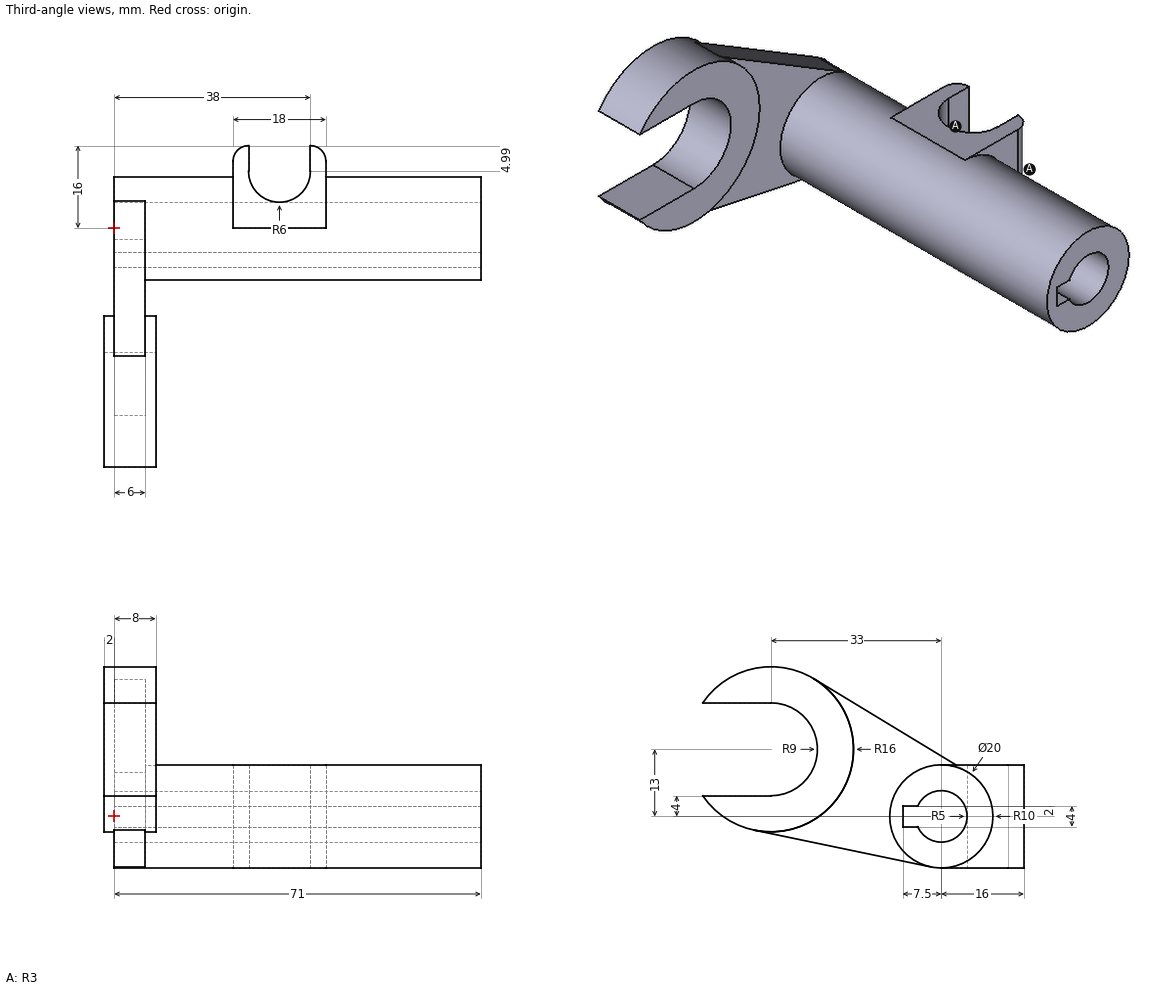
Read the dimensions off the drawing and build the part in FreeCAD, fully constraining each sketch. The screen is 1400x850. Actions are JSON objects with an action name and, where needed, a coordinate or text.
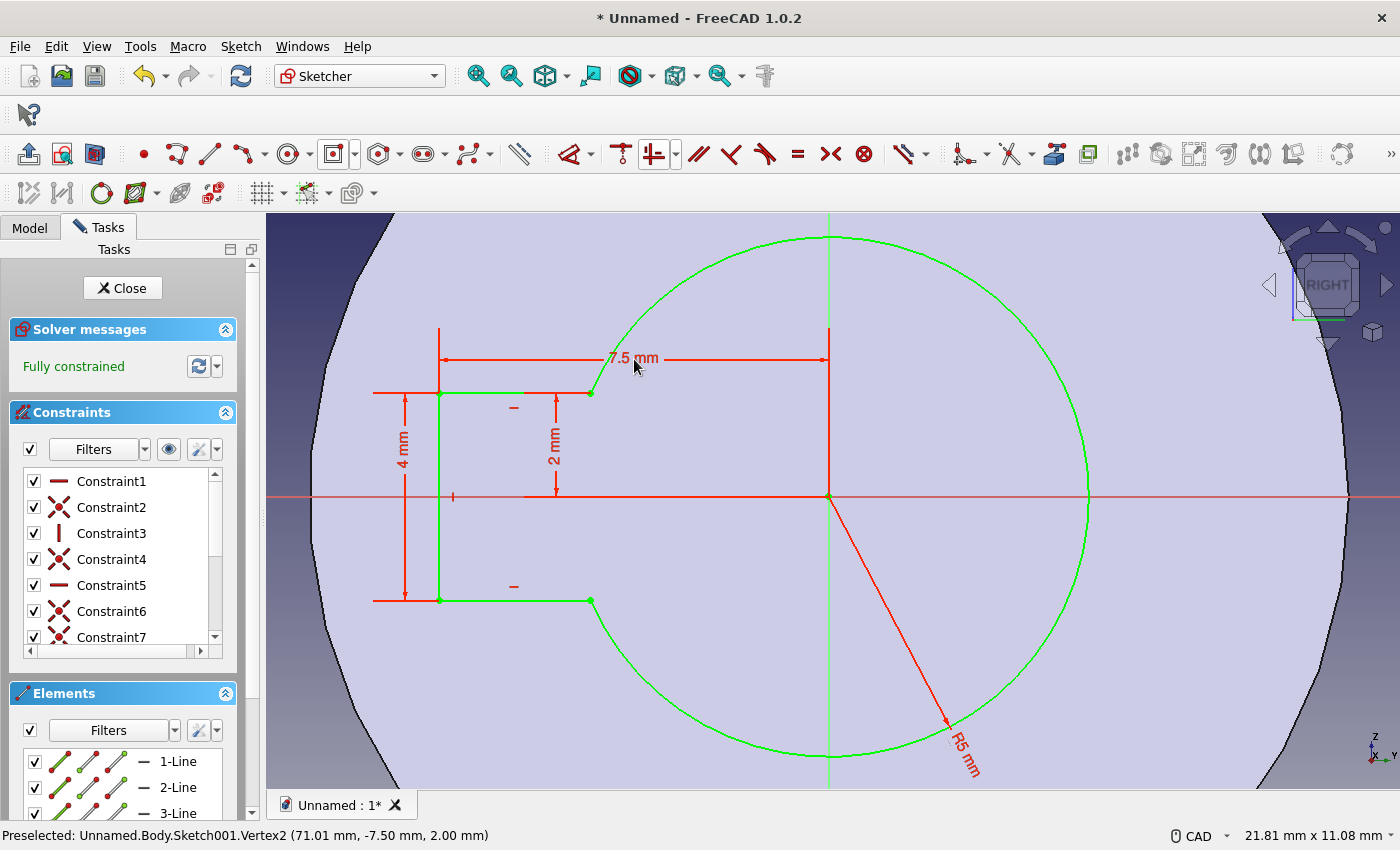
{"action": "left_click", "coordinate": [123, 288]}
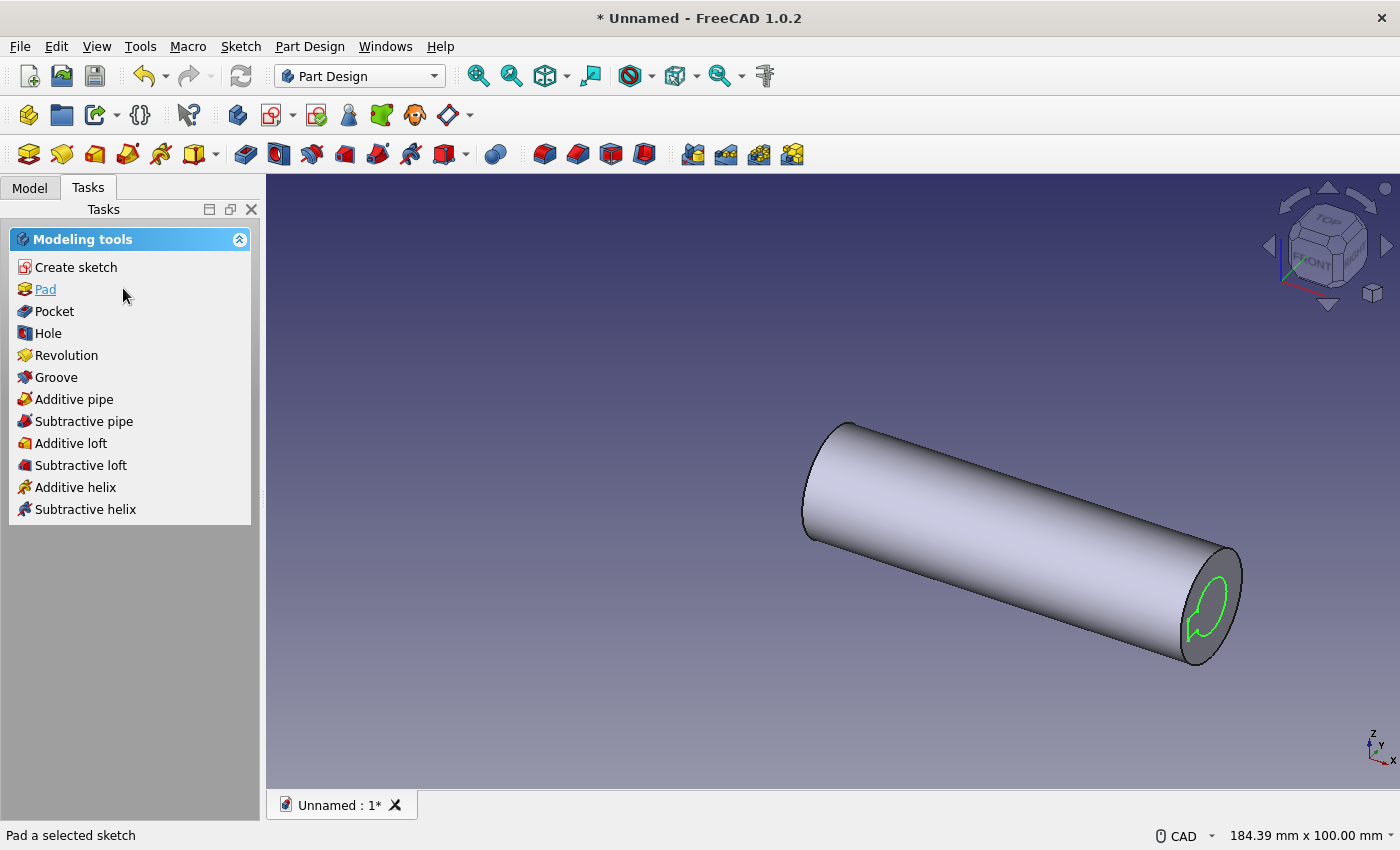
{"action": "left_click", "coordinate": [246, 154]}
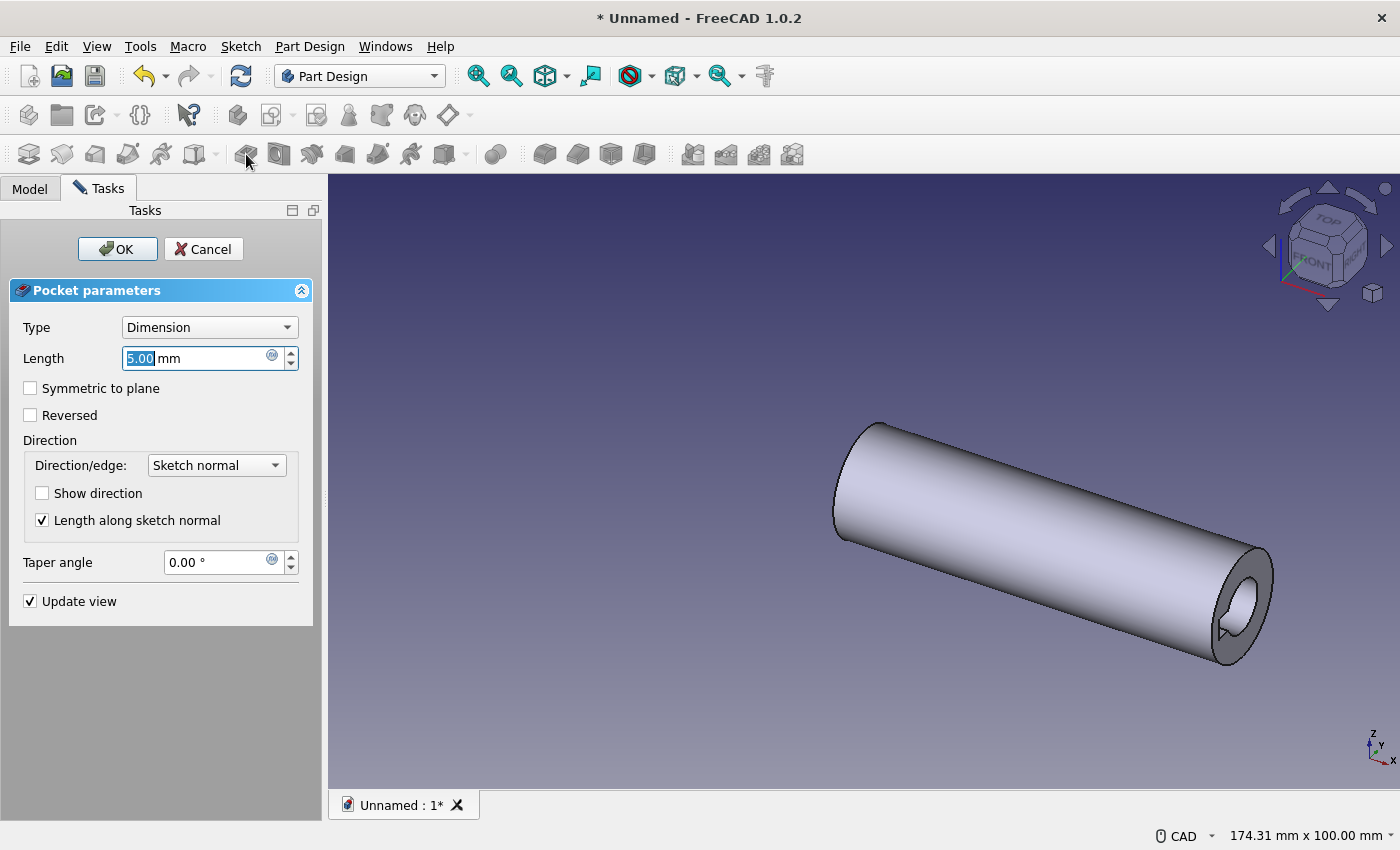
{"action": "left_click", "coordinate": [210, 328]}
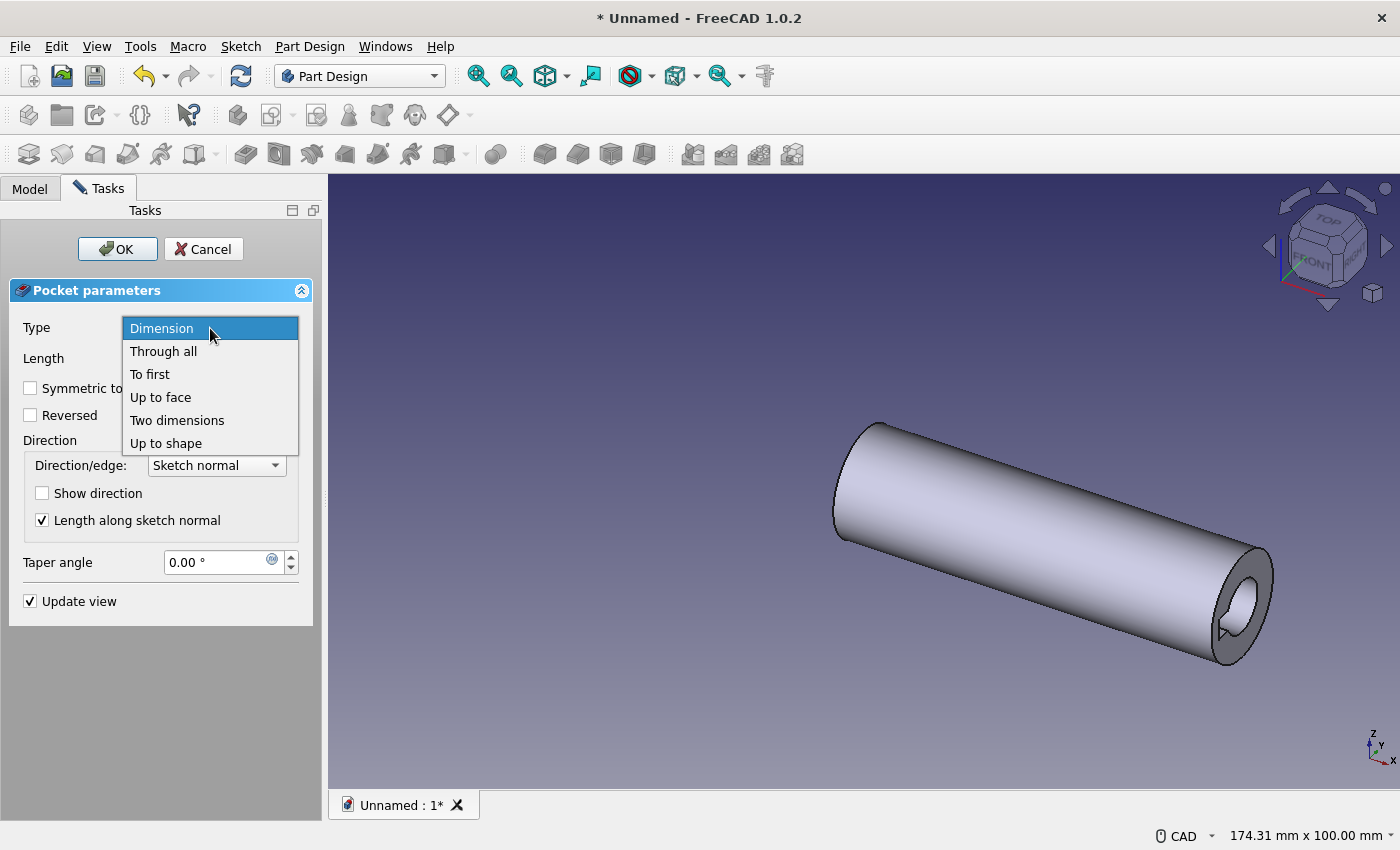
{"action": "left_click", "coordinate": [208, 374]}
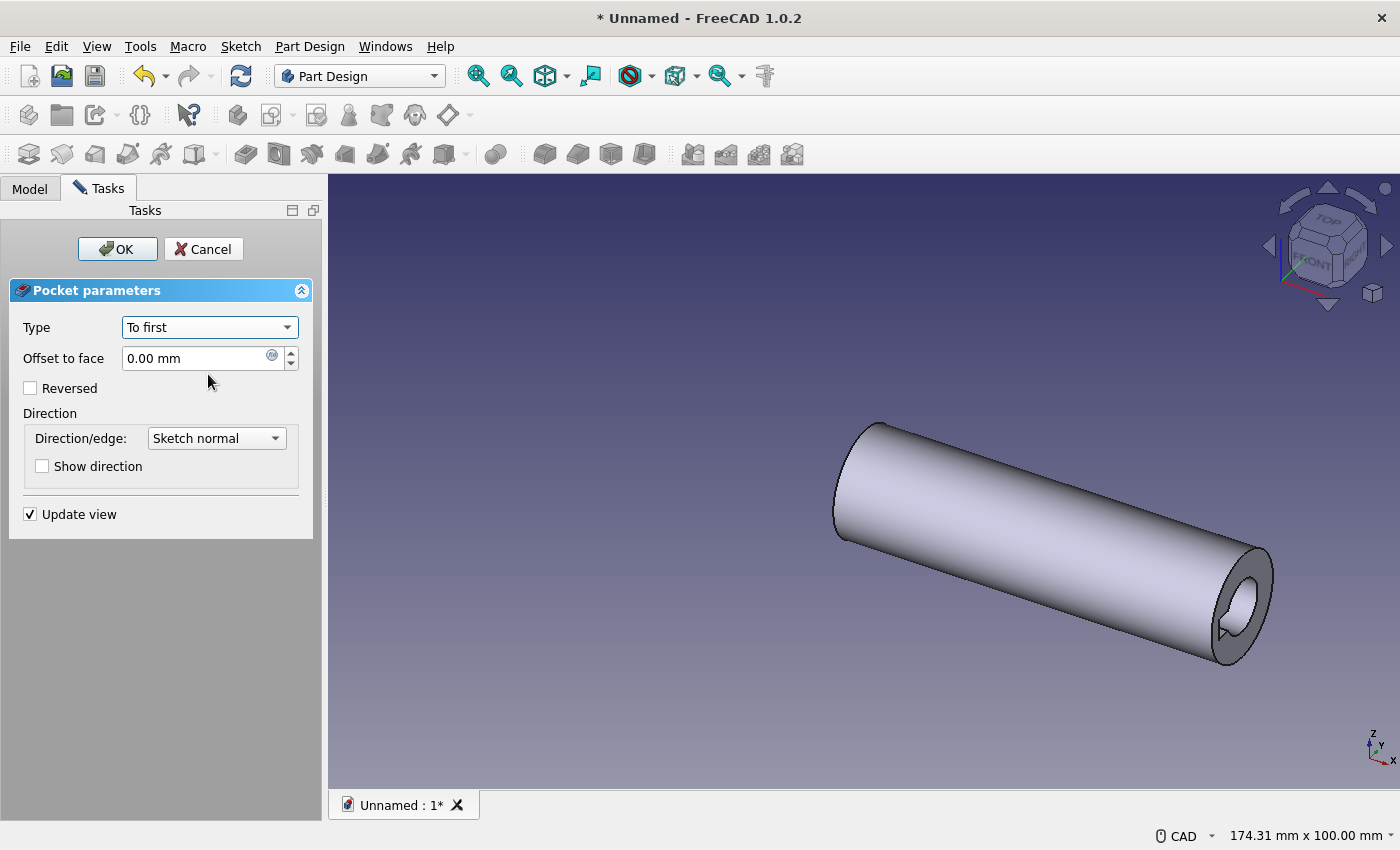
{"action": "left_click", "coordinate": [118, 249]}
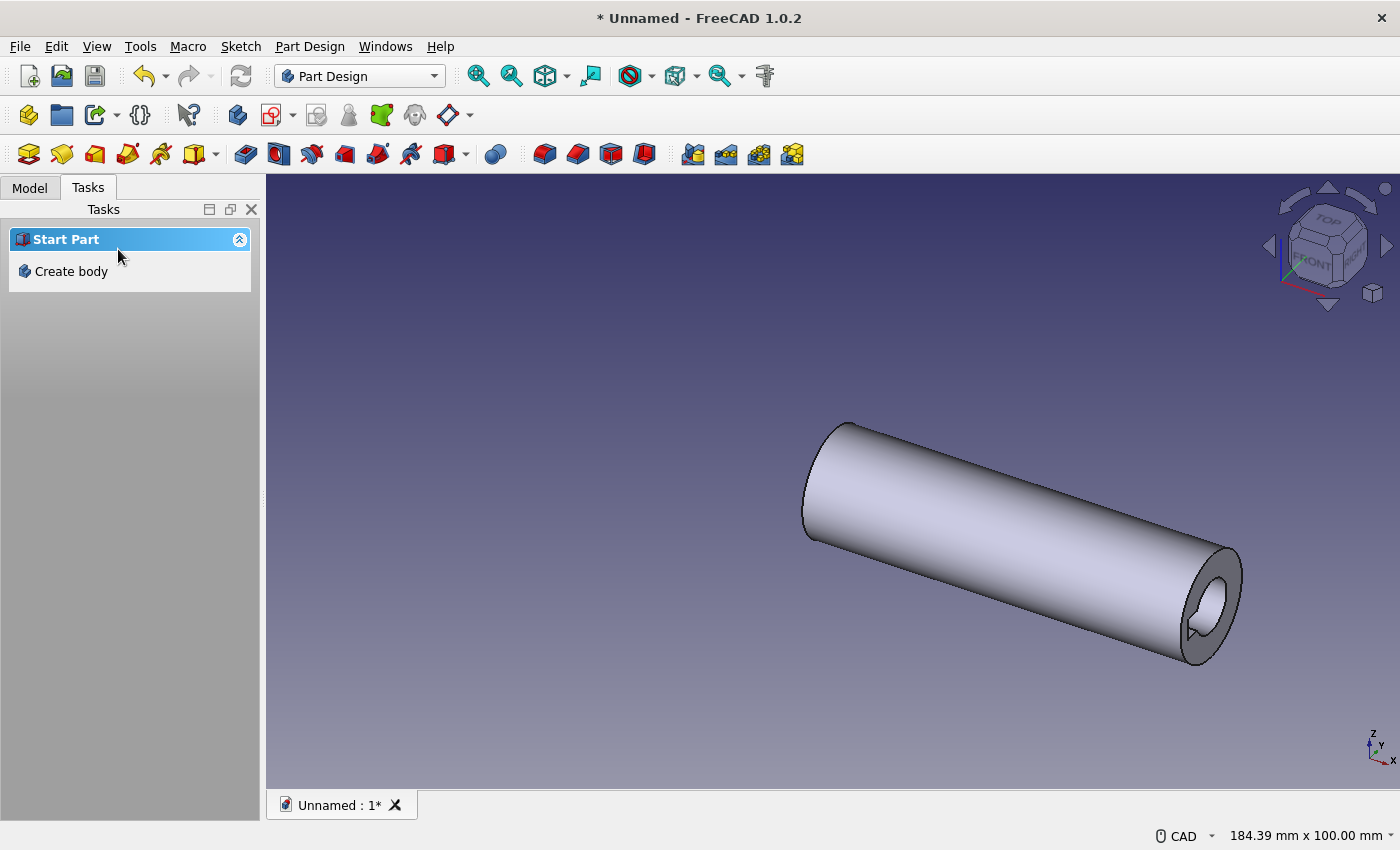
{"action": "left_click", "coordinate": [30, 188]}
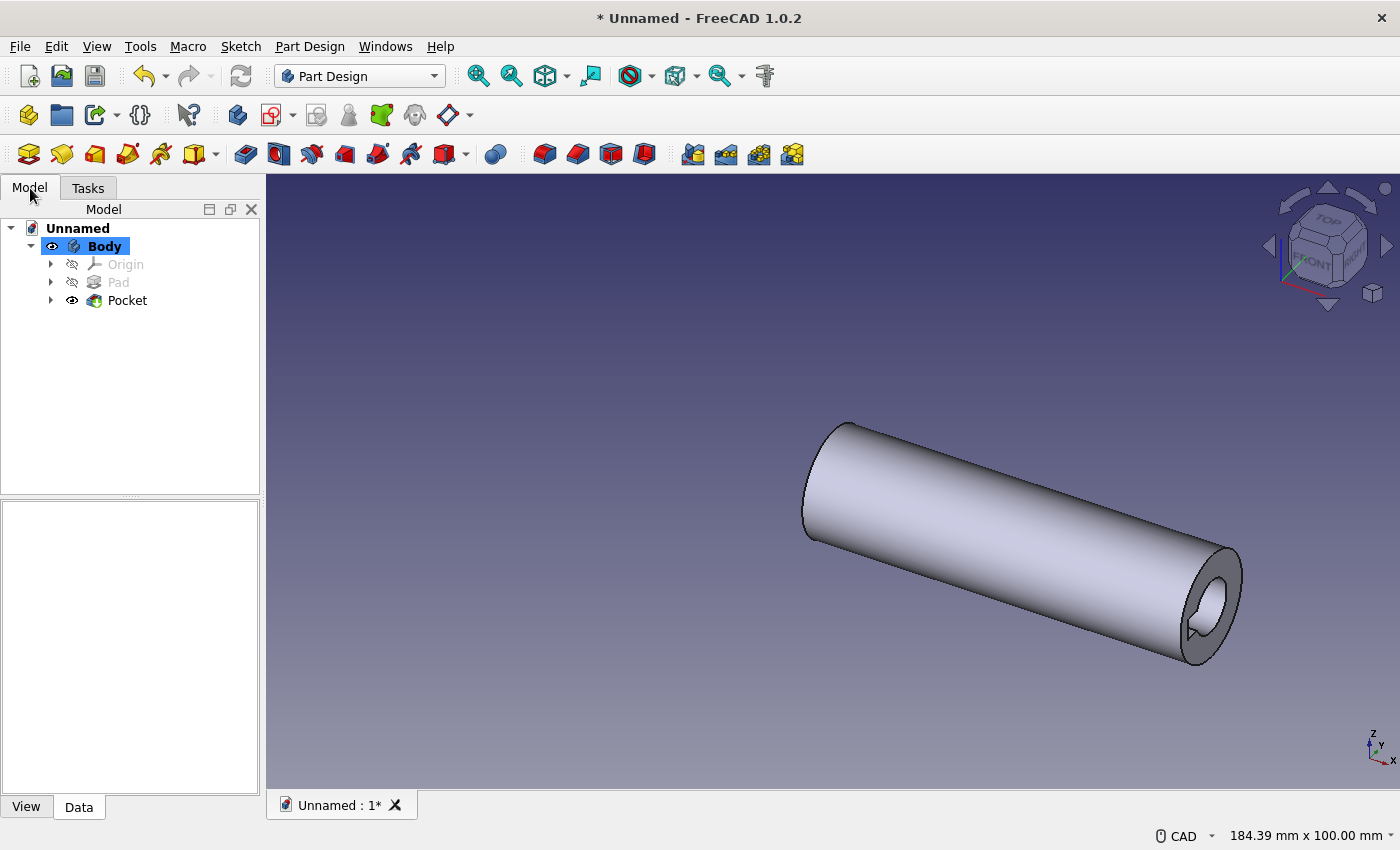
{"action": "left_click", "coordinate": [51, 264]}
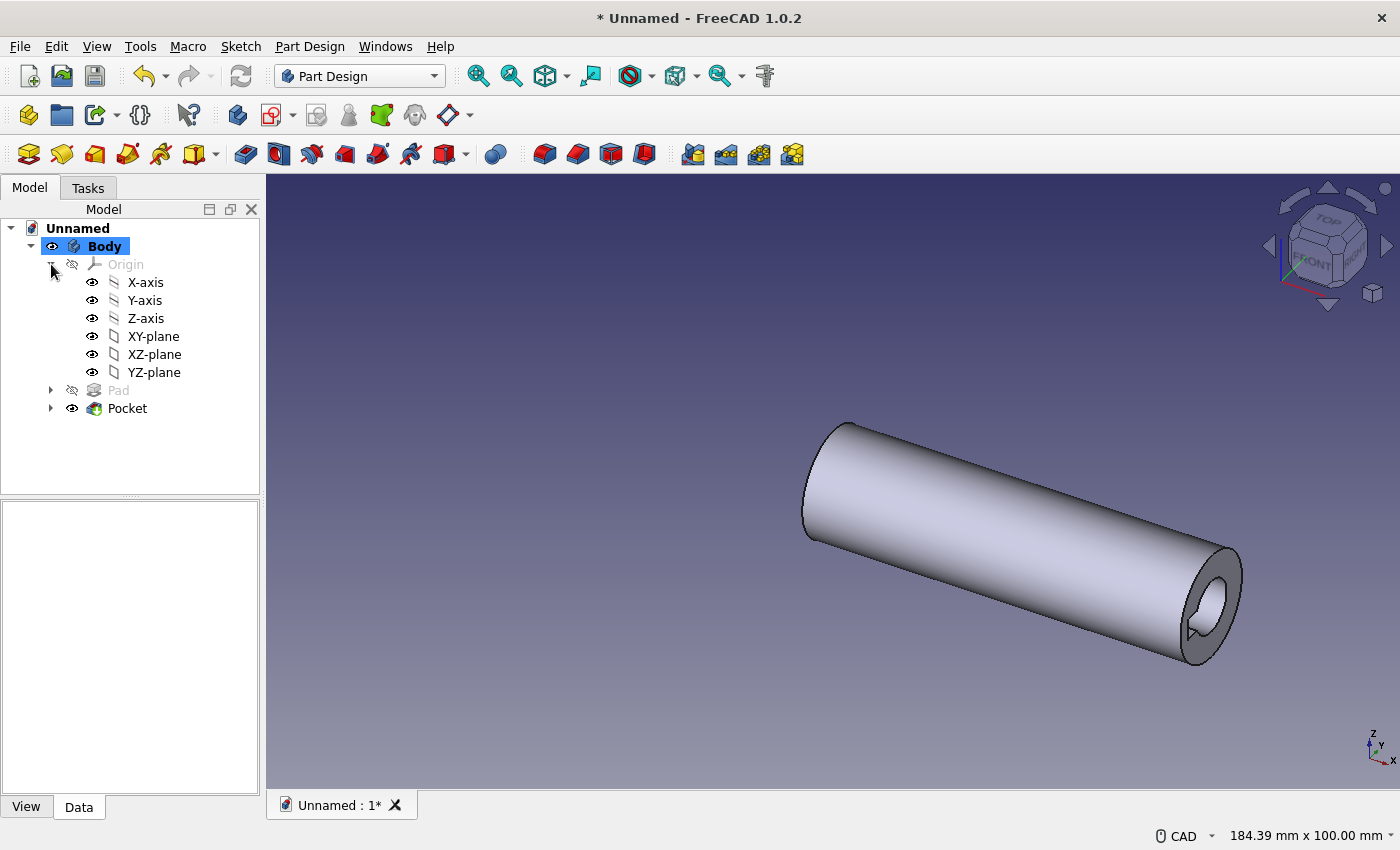
{"action": "left_click", "coordinate": [137, 372]}